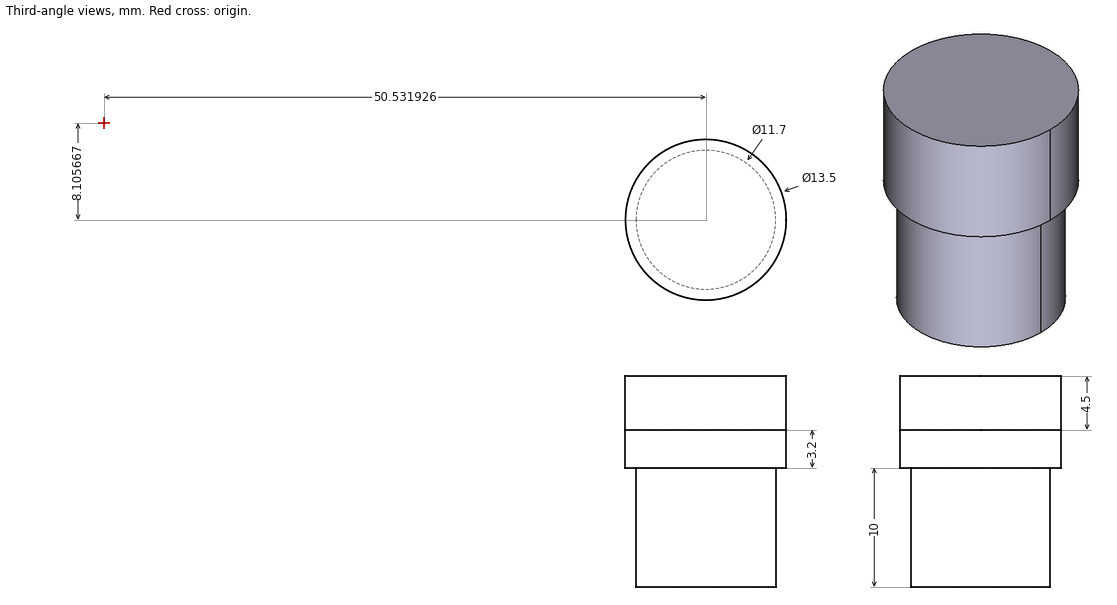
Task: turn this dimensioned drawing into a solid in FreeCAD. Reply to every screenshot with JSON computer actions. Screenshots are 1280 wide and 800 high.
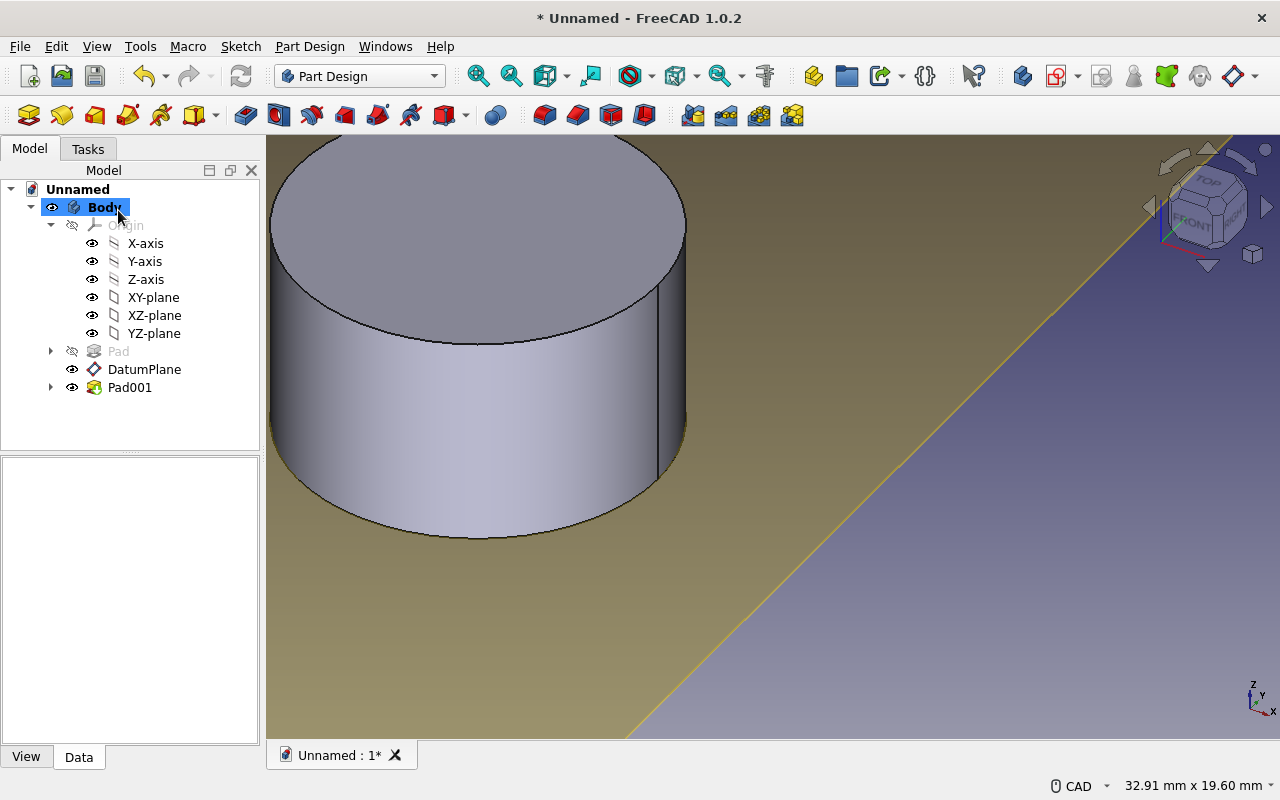
{"action": "left_click", "coordinate": [117, 369]}
{"action": "key", "text": "space"}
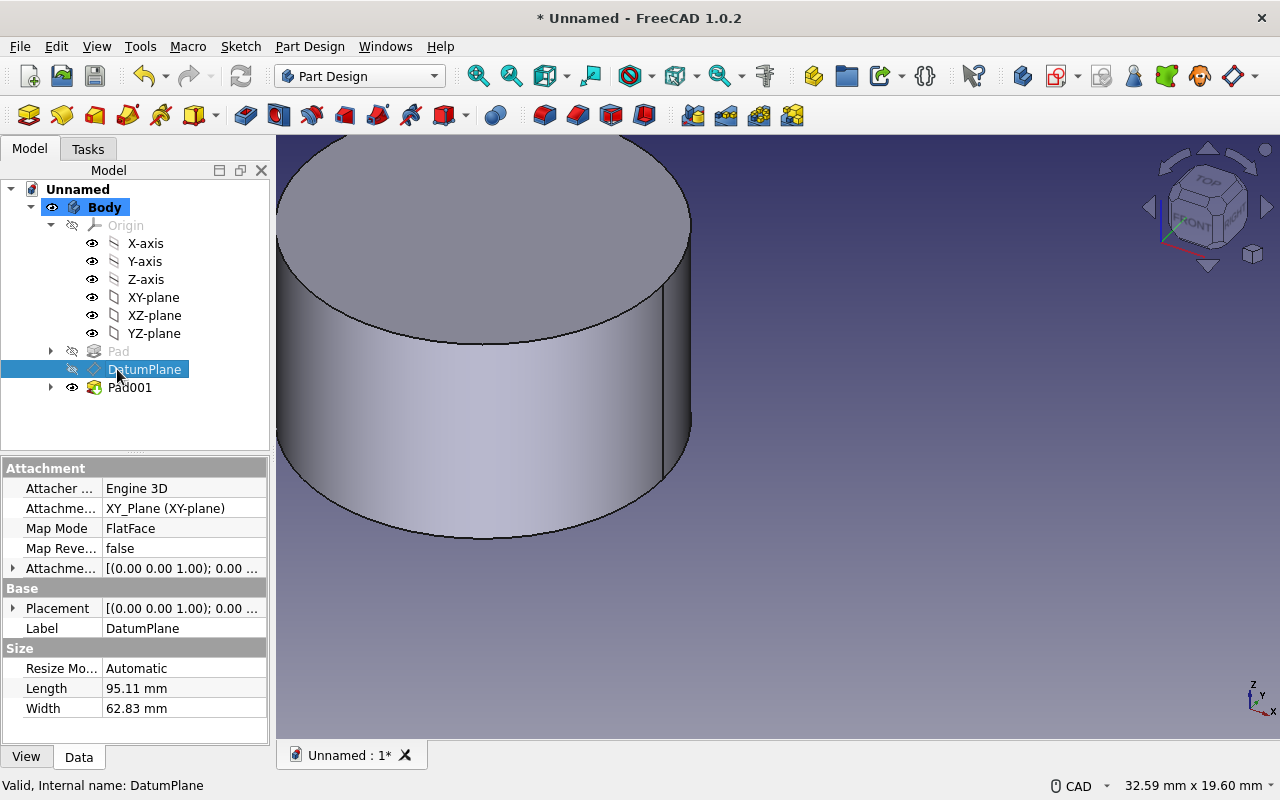
{"action": "key", "text": "v f"}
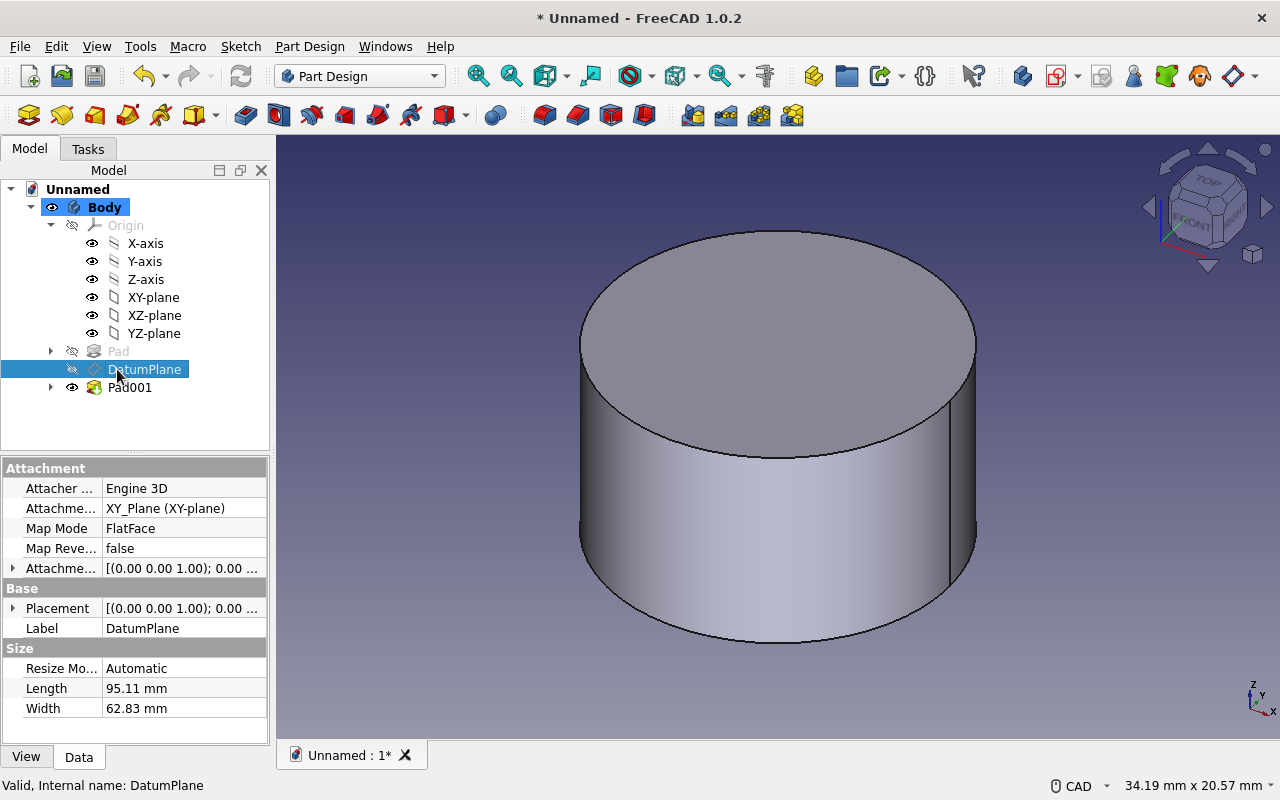
{"action": "key", "text": "5"}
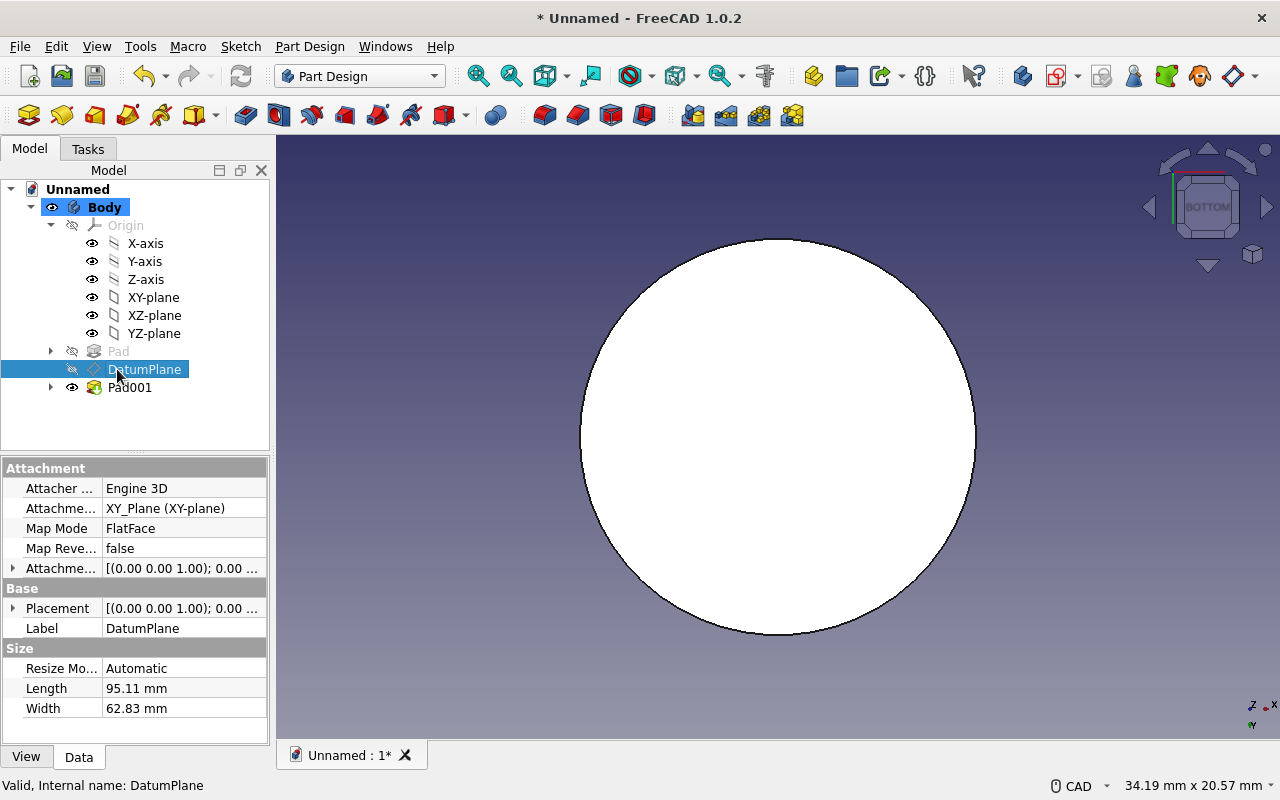
{"action": "left_click", "coordinate": [778, 436]}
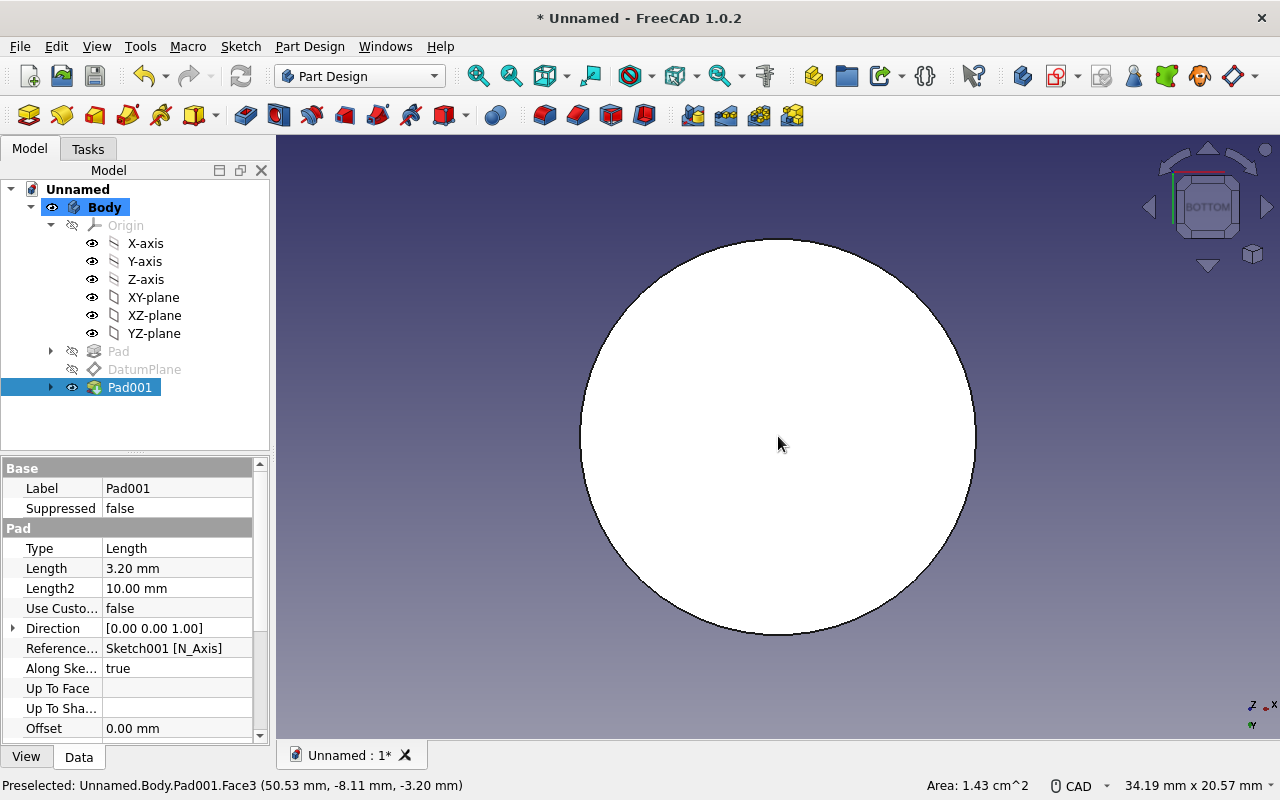
{"action": "left_click", "coordinate": [1056, 76]}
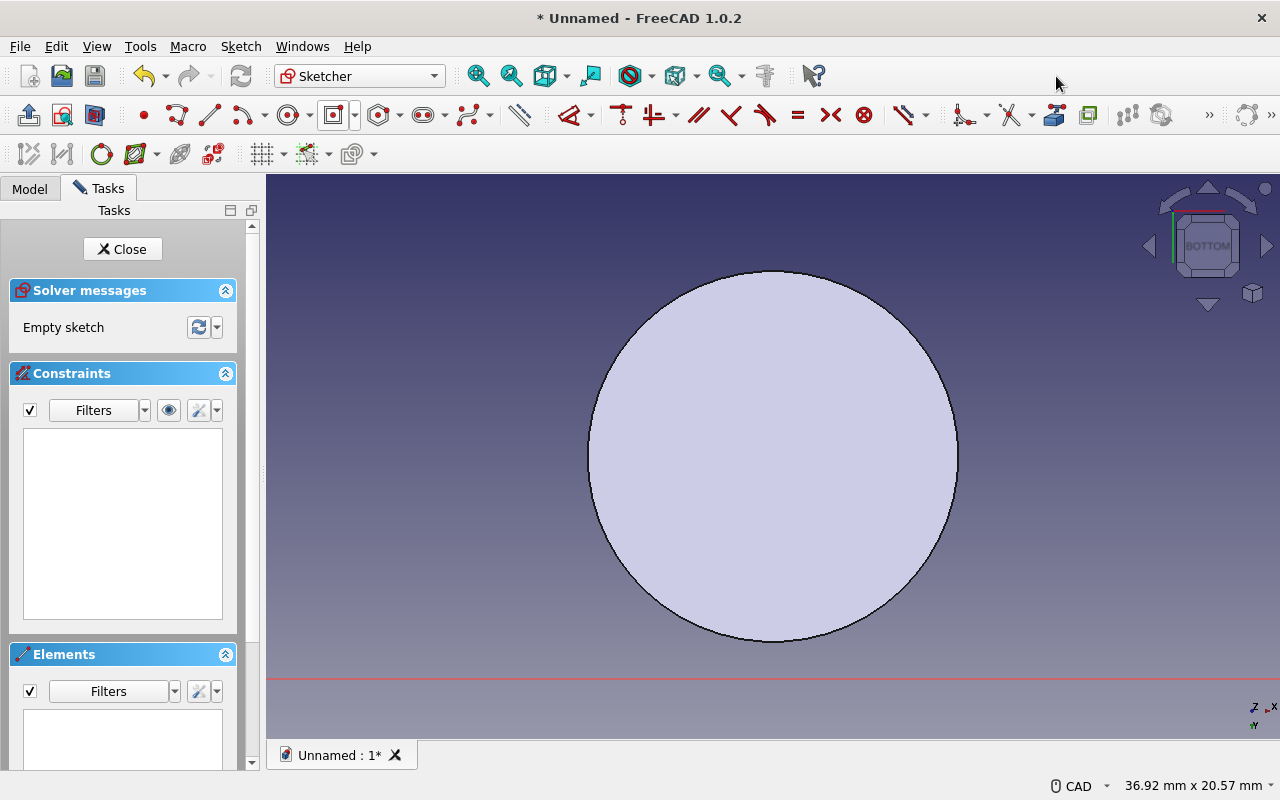
{"action": "key", "text": "g c"}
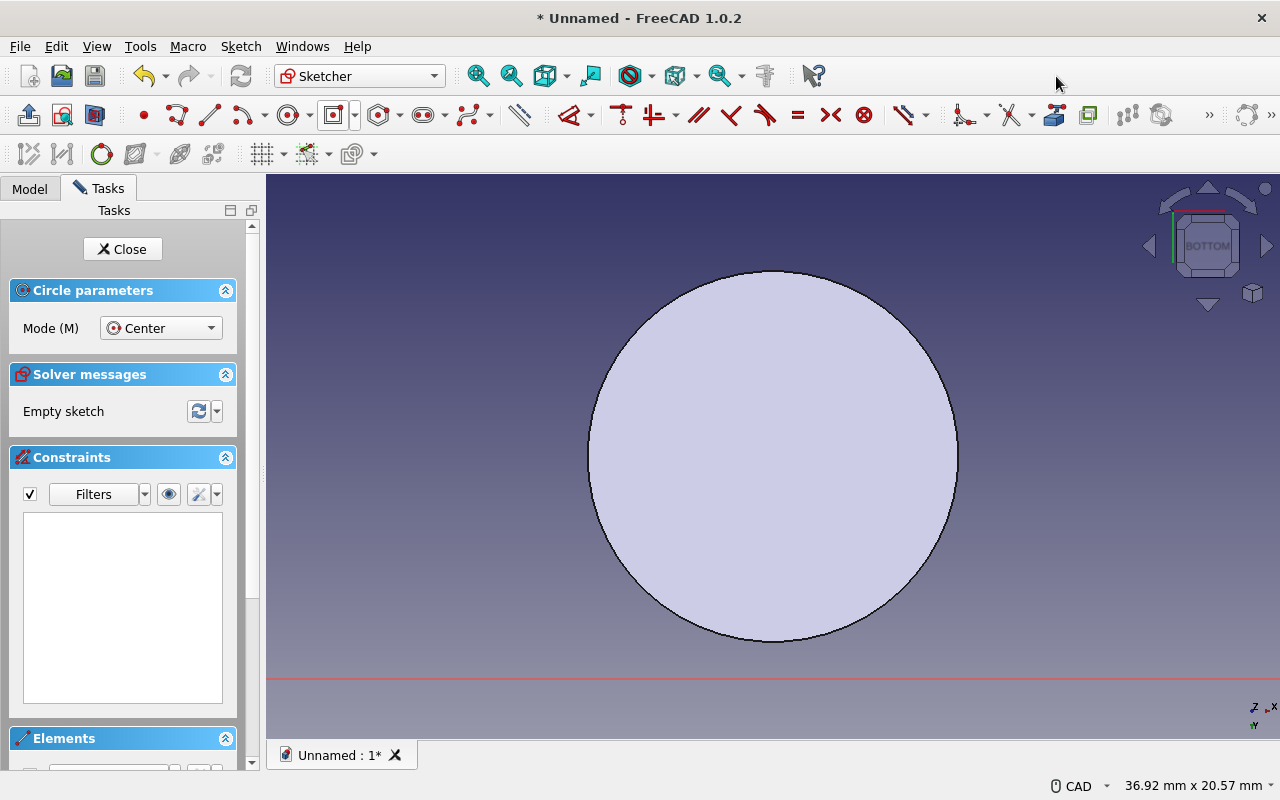
{"action": "left_click", "coordinate": [773, 457]}
{"action": "mouse_move", "coordinate": [887, 343]}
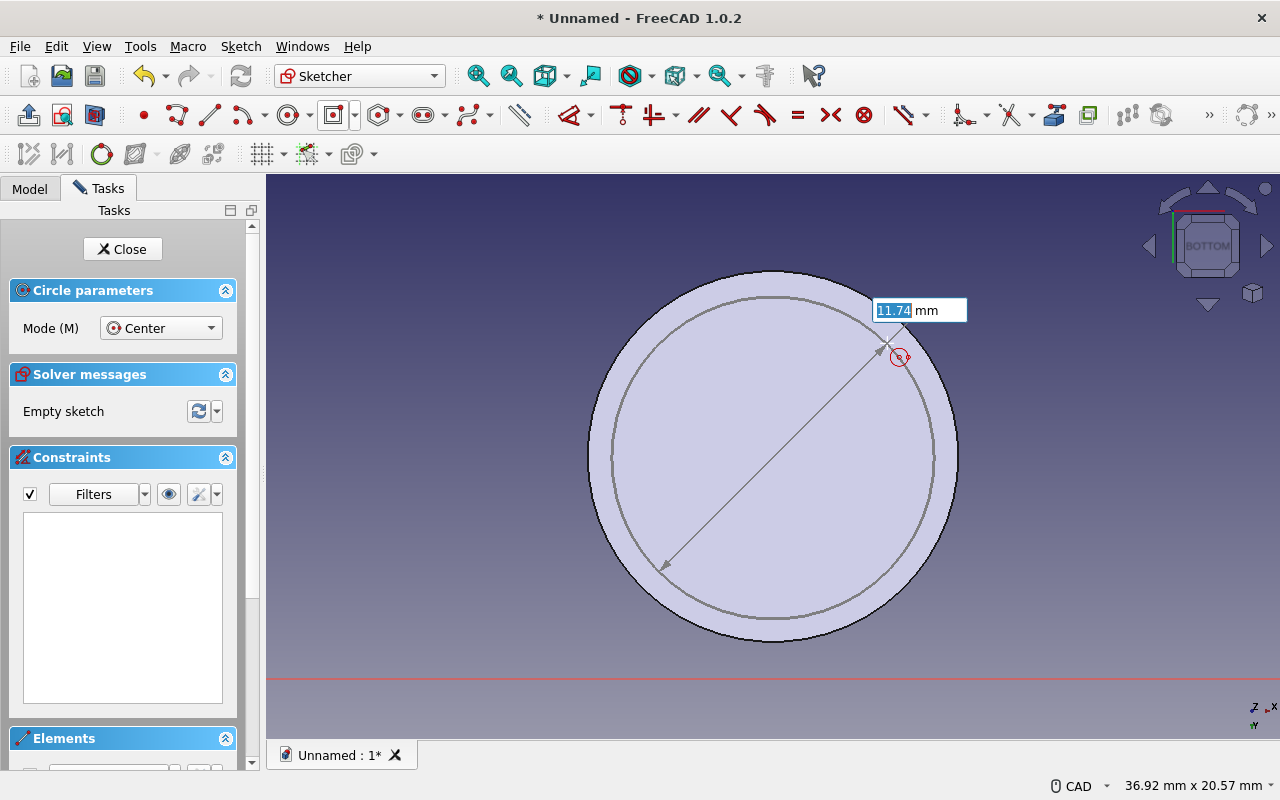
{"action": "type", "text": "11.7"}
{"action": "key", "text": "Return"}
{"action": "key", "text": "Escape"}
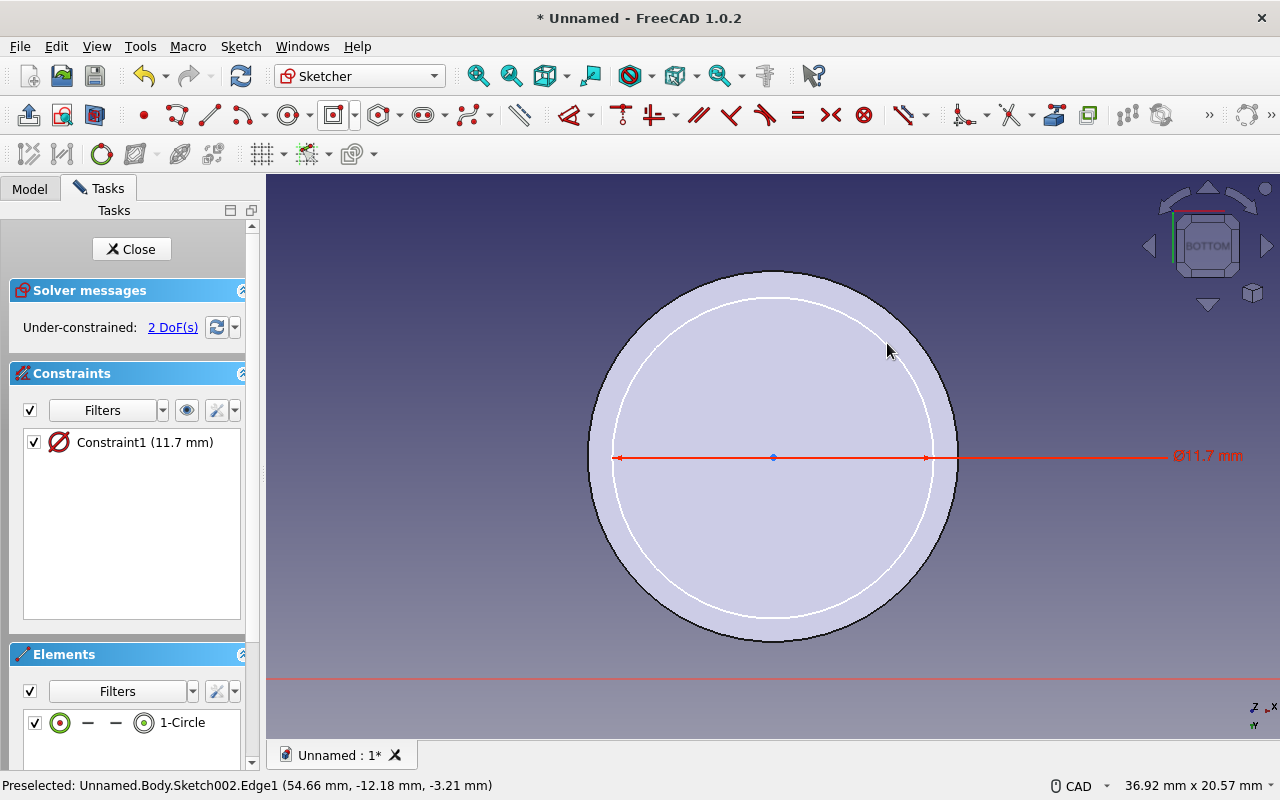
{"action": "key", "text": "d"}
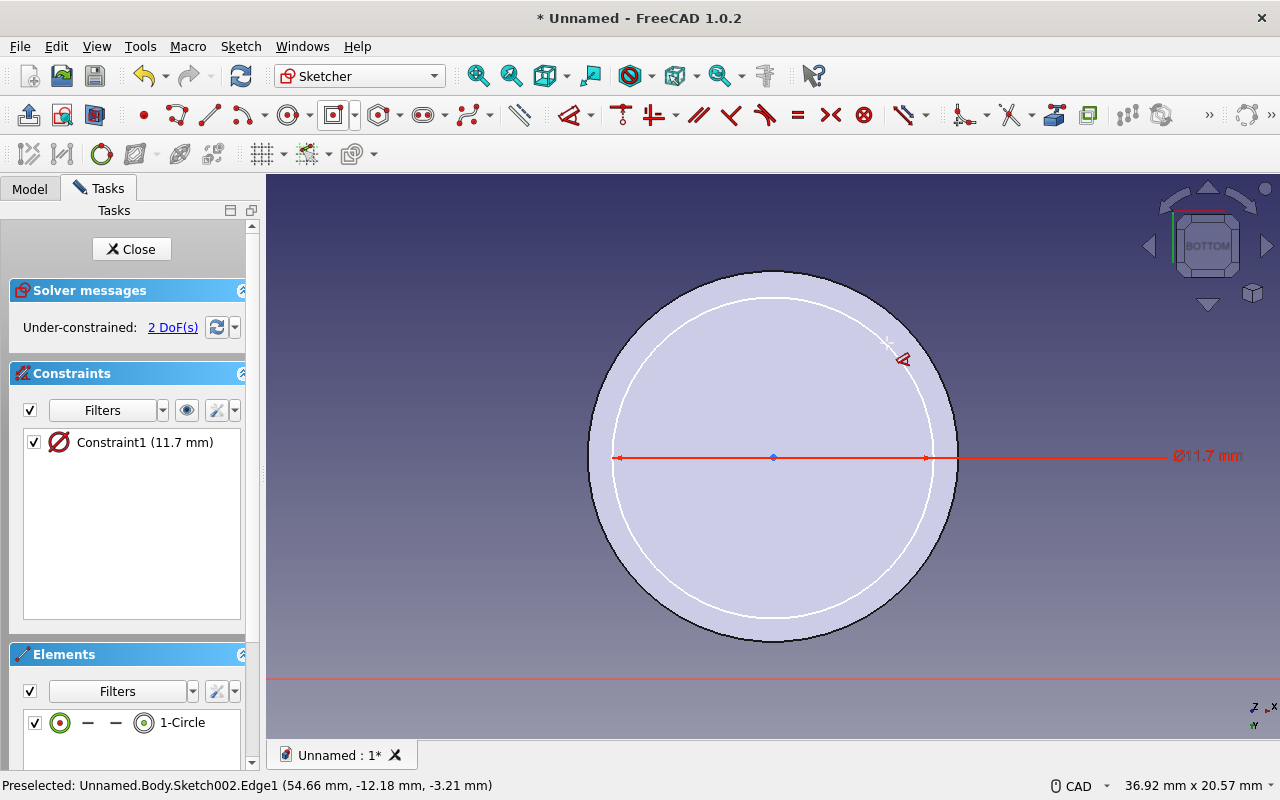
{"action": "left_click", "coordinate": [773, 458]}
{"action": "left_click", "coordinate": [807, 569]}